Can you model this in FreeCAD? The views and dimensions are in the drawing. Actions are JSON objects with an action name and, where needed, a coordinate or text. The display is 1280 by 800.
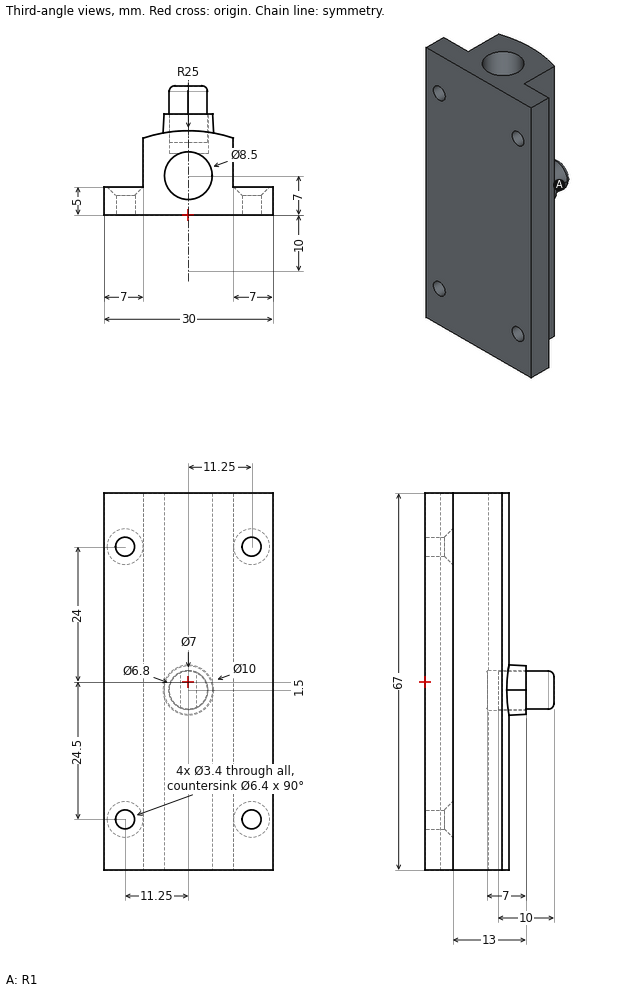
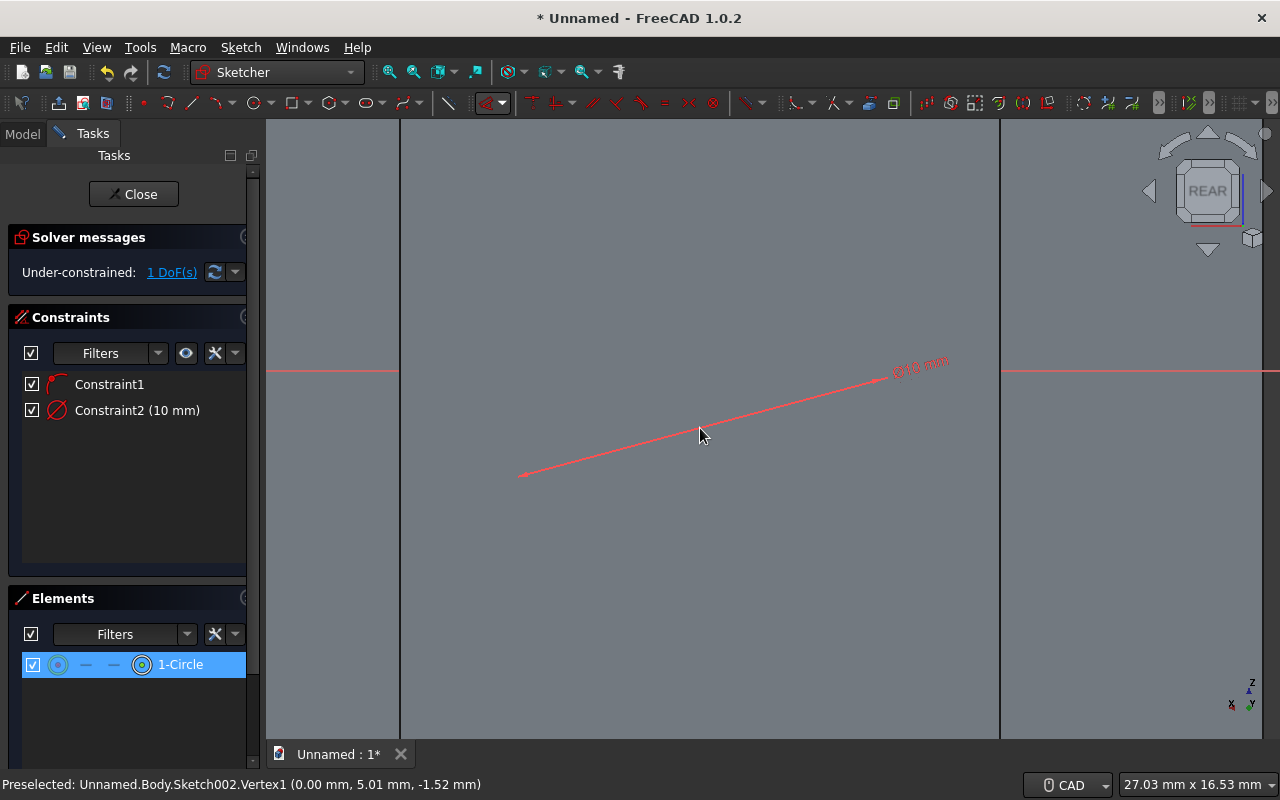
{"action": "key", "text": "i"}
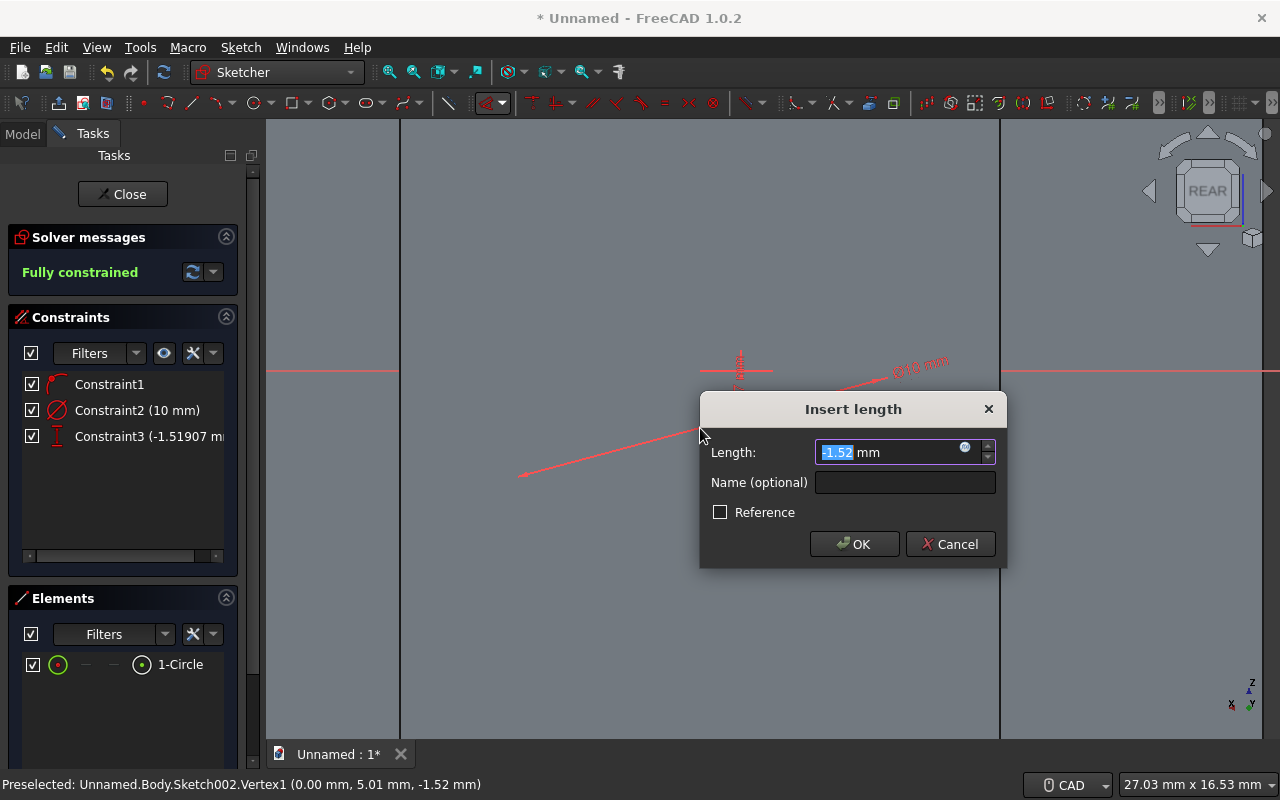
{"action": "type", "text": "-1.5"}
{"action": "key", "text": "Return"}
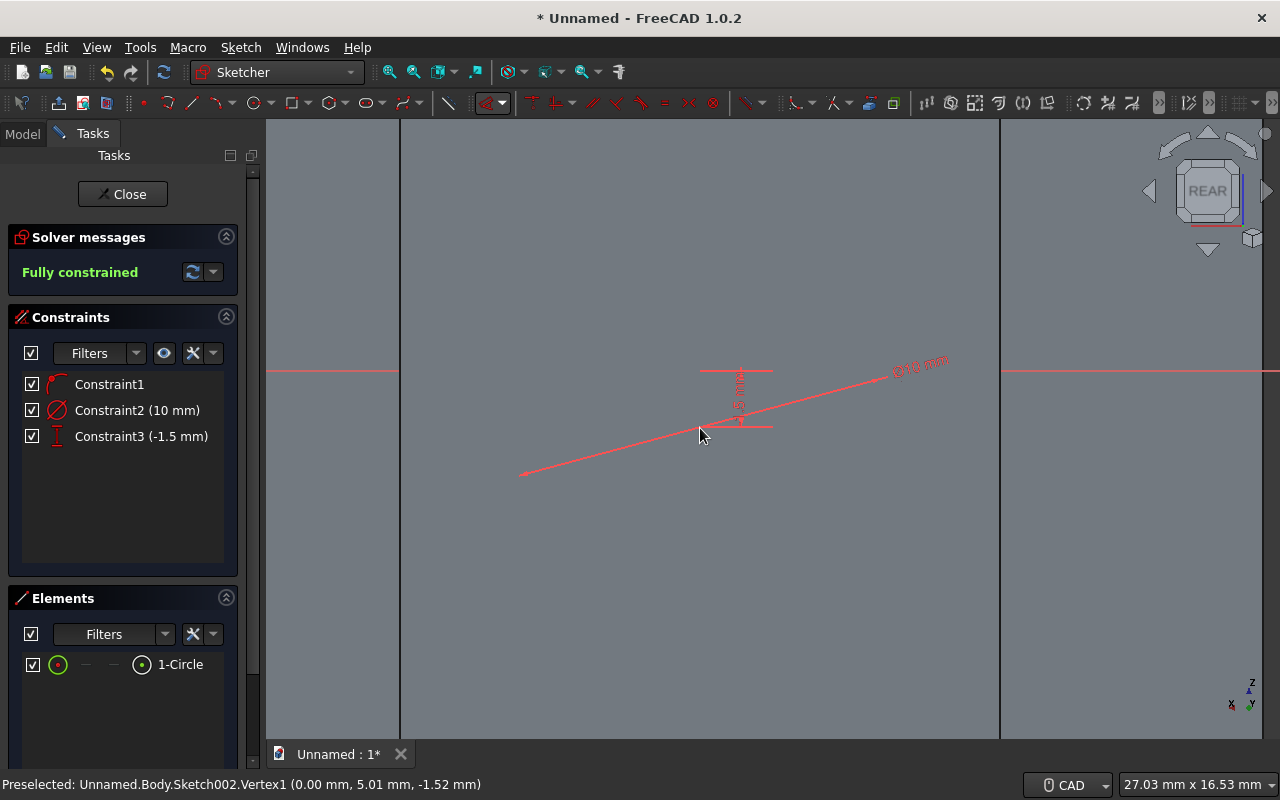
{"action": "left_click", "coordinate": [123, 194]}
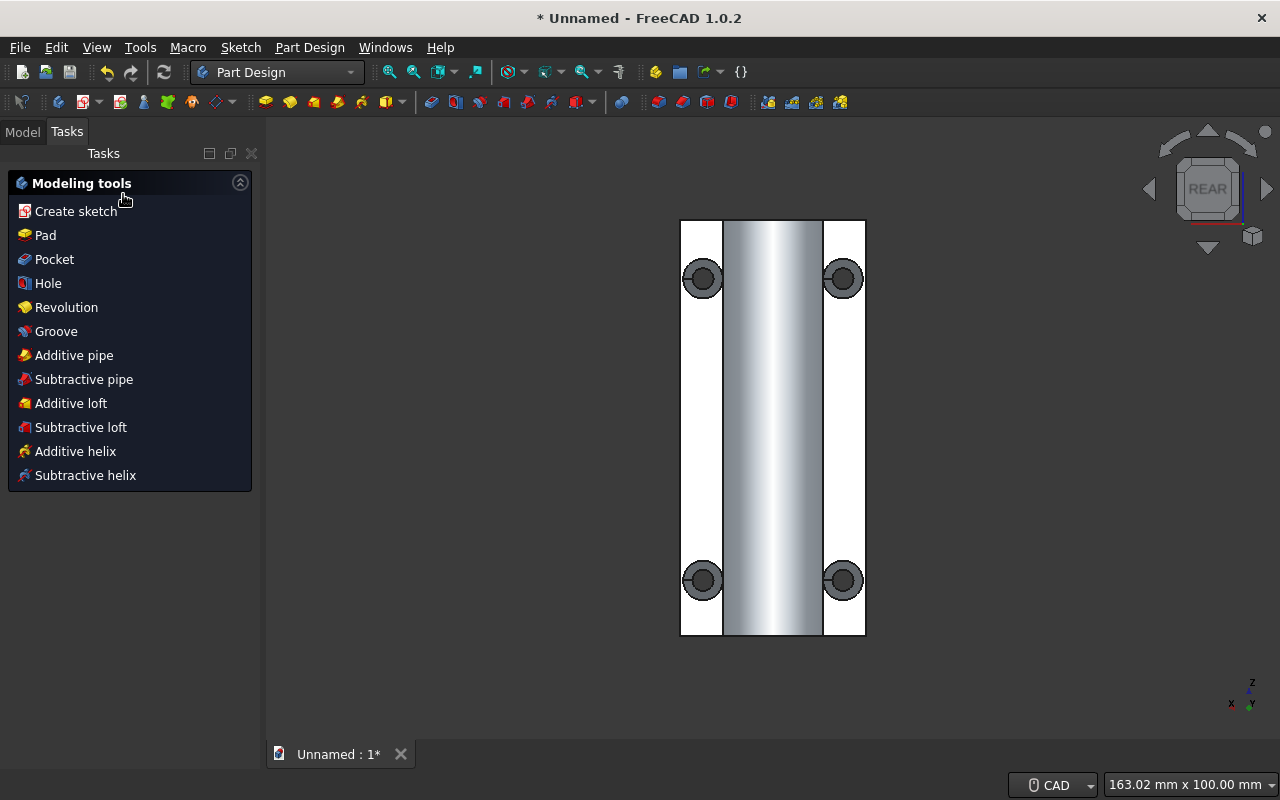
{"action": "left_click", "coordinate": [266, 102]}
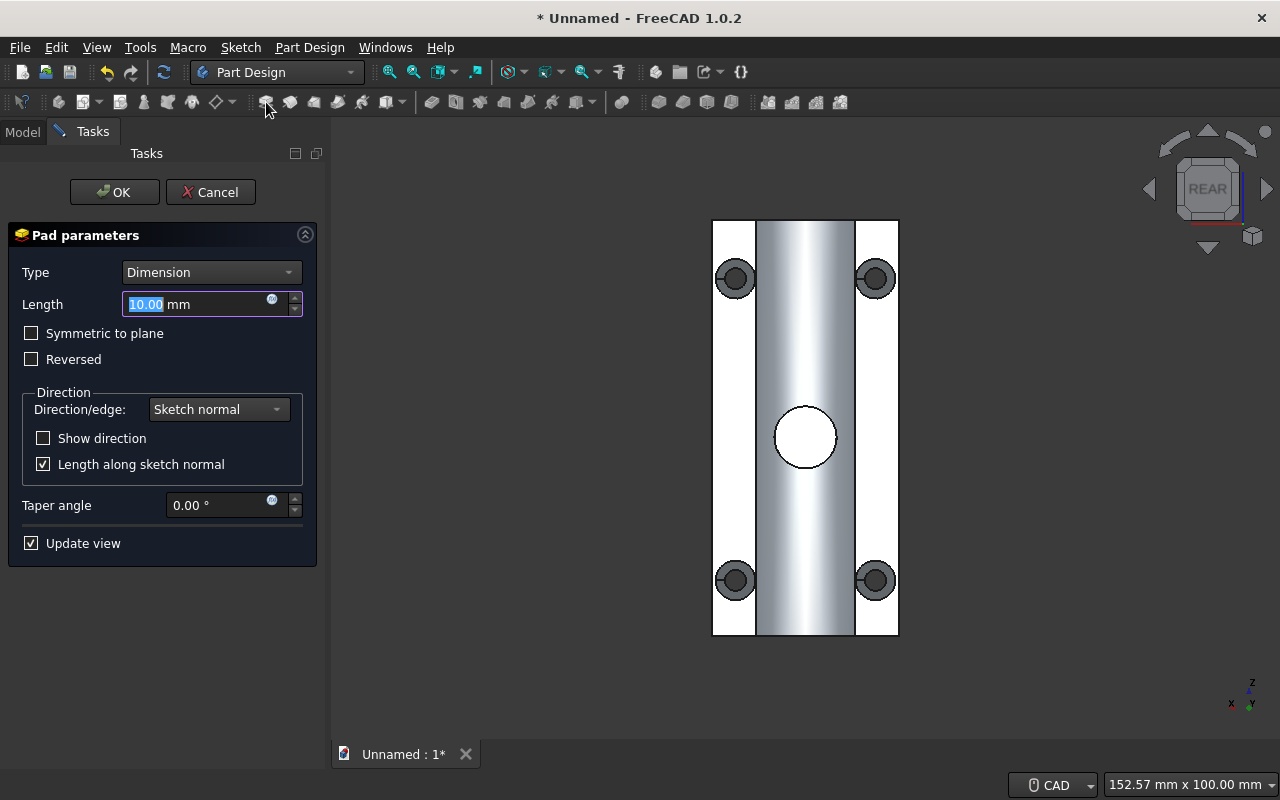
{"action": "type", "text": "13"}
{"action": "key", "text": "Tab"}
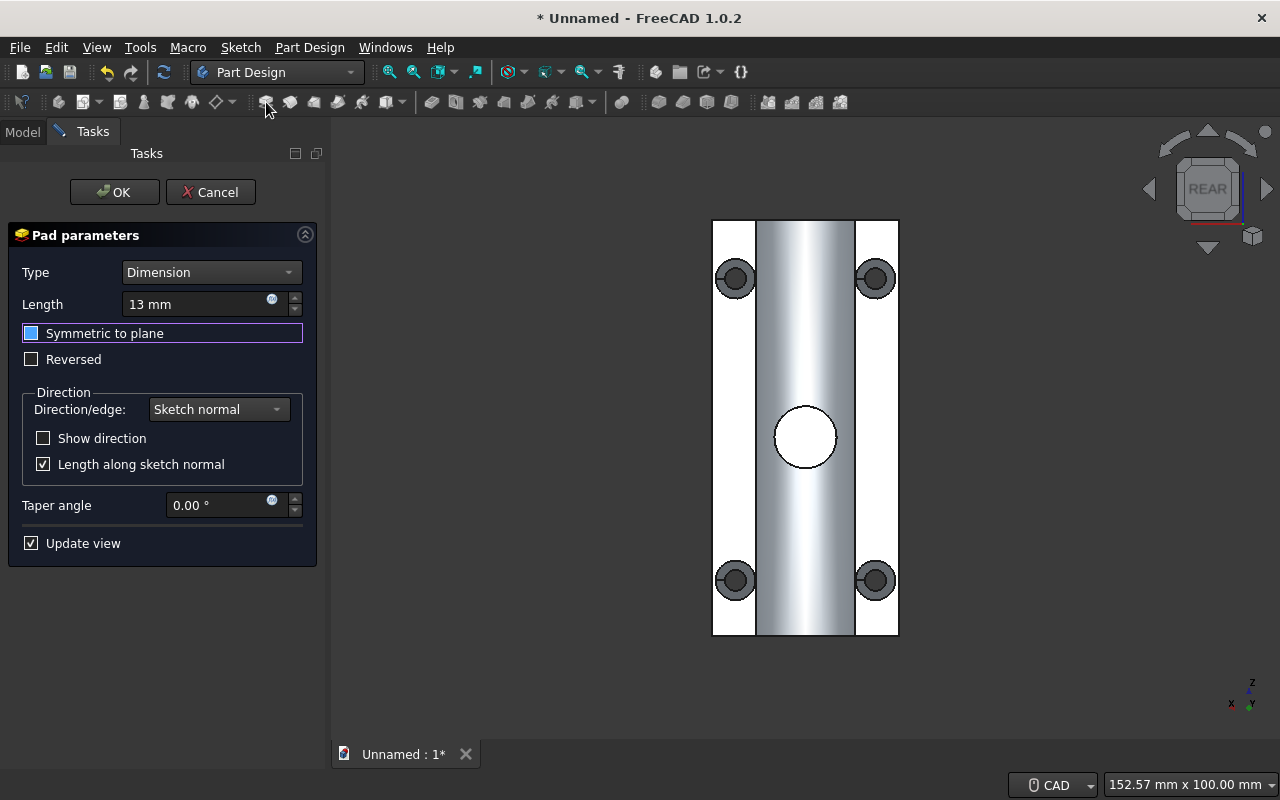
{"action": "triple_click", "coordinate": [226, 505]}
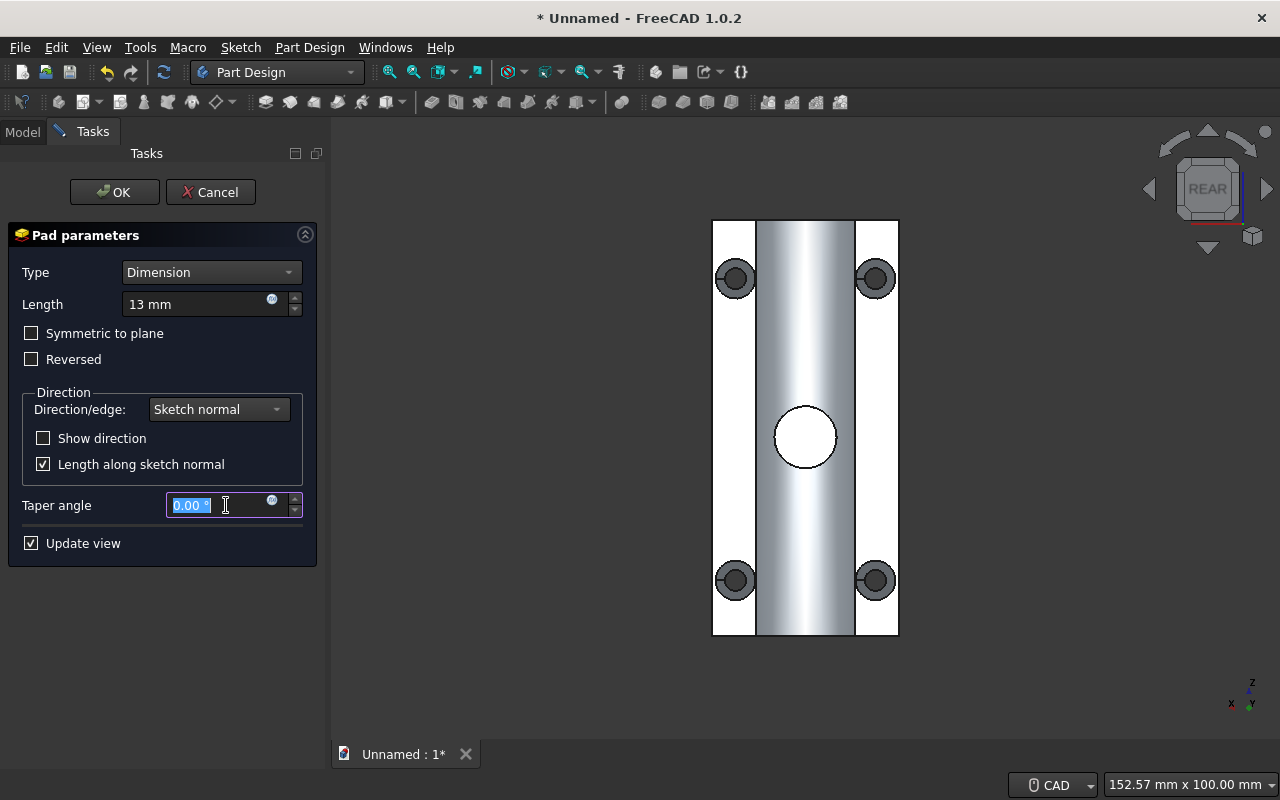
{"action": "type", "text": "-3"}
{"action": "key", "text": "Tab"}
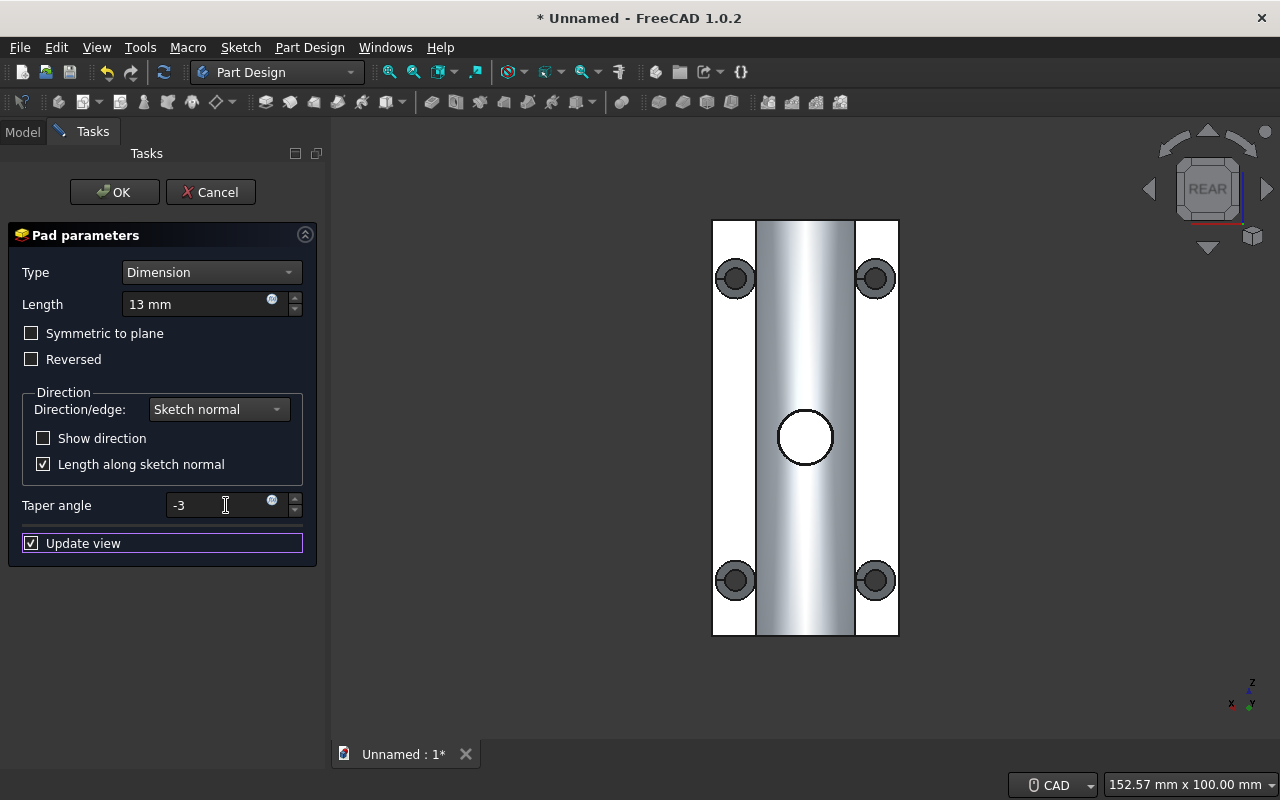
{"action": "left_click", "coordinate": [115, 192]}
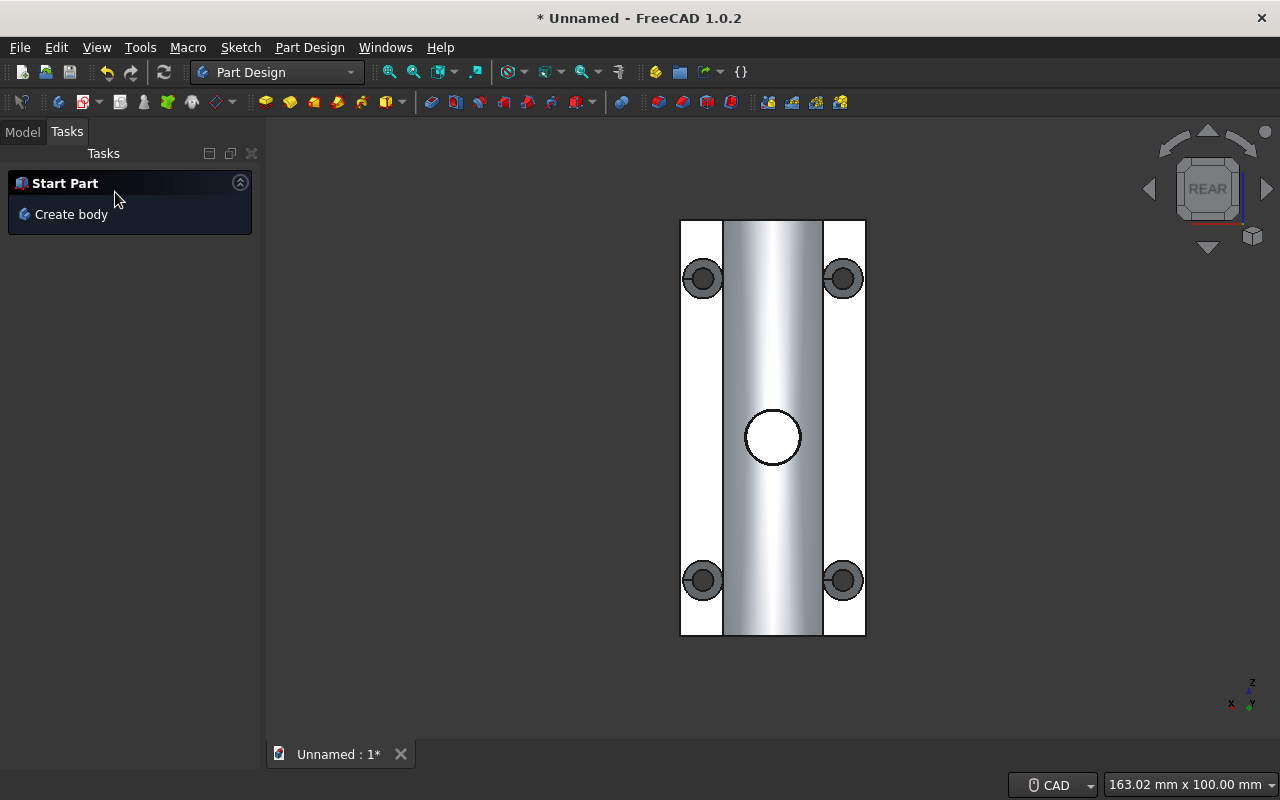
{"action": "left_click", "coordinate": [773, 436]}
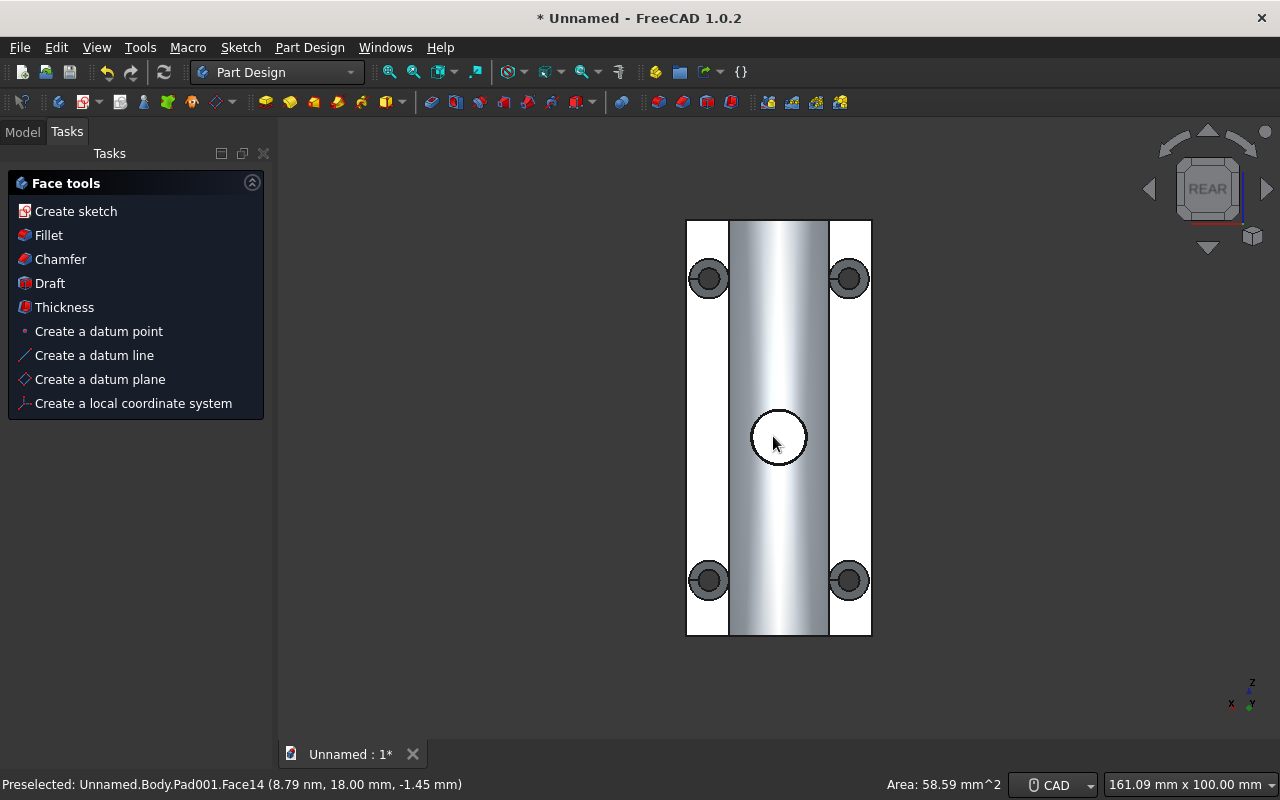
{"action": "left_click", "coordinate": [84, 102]}